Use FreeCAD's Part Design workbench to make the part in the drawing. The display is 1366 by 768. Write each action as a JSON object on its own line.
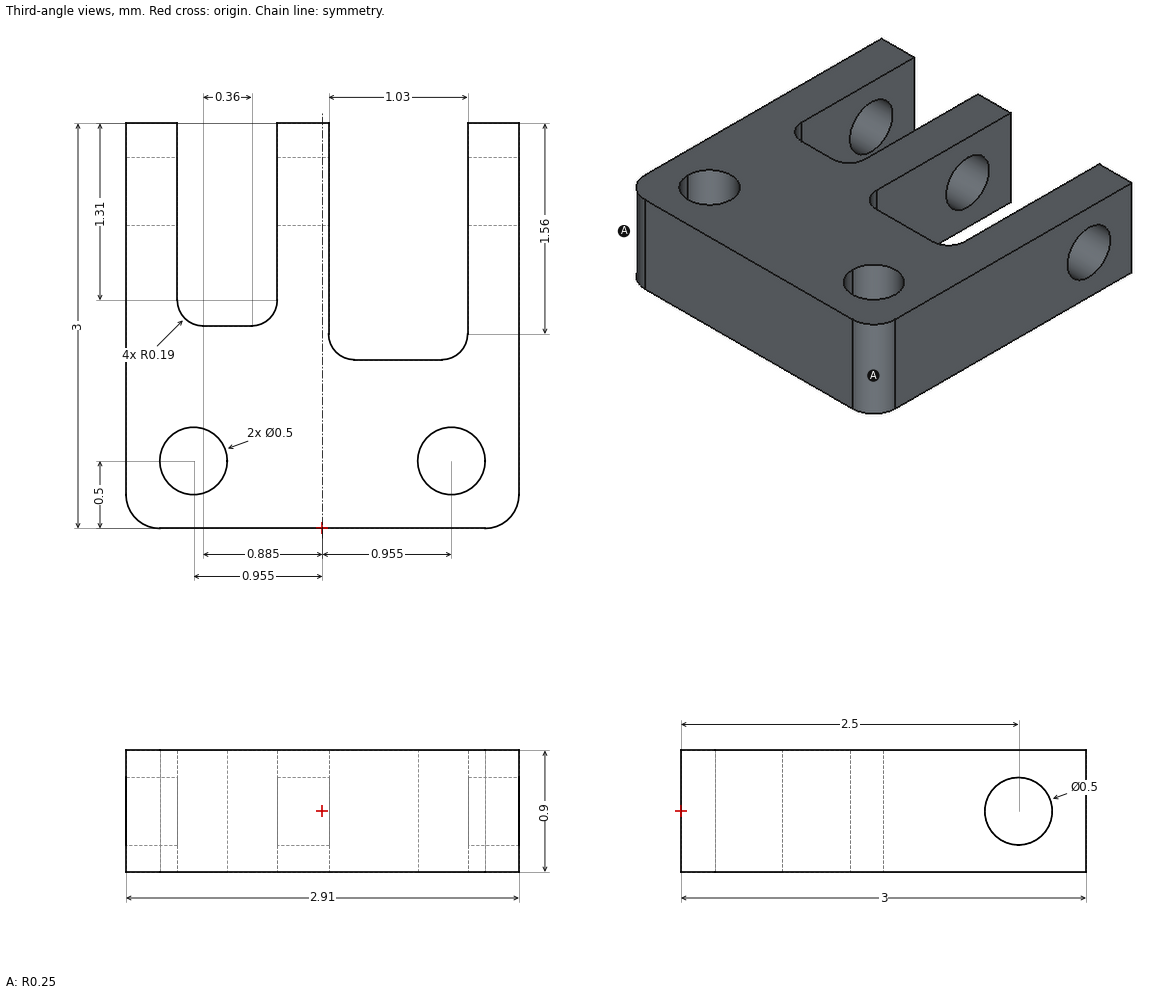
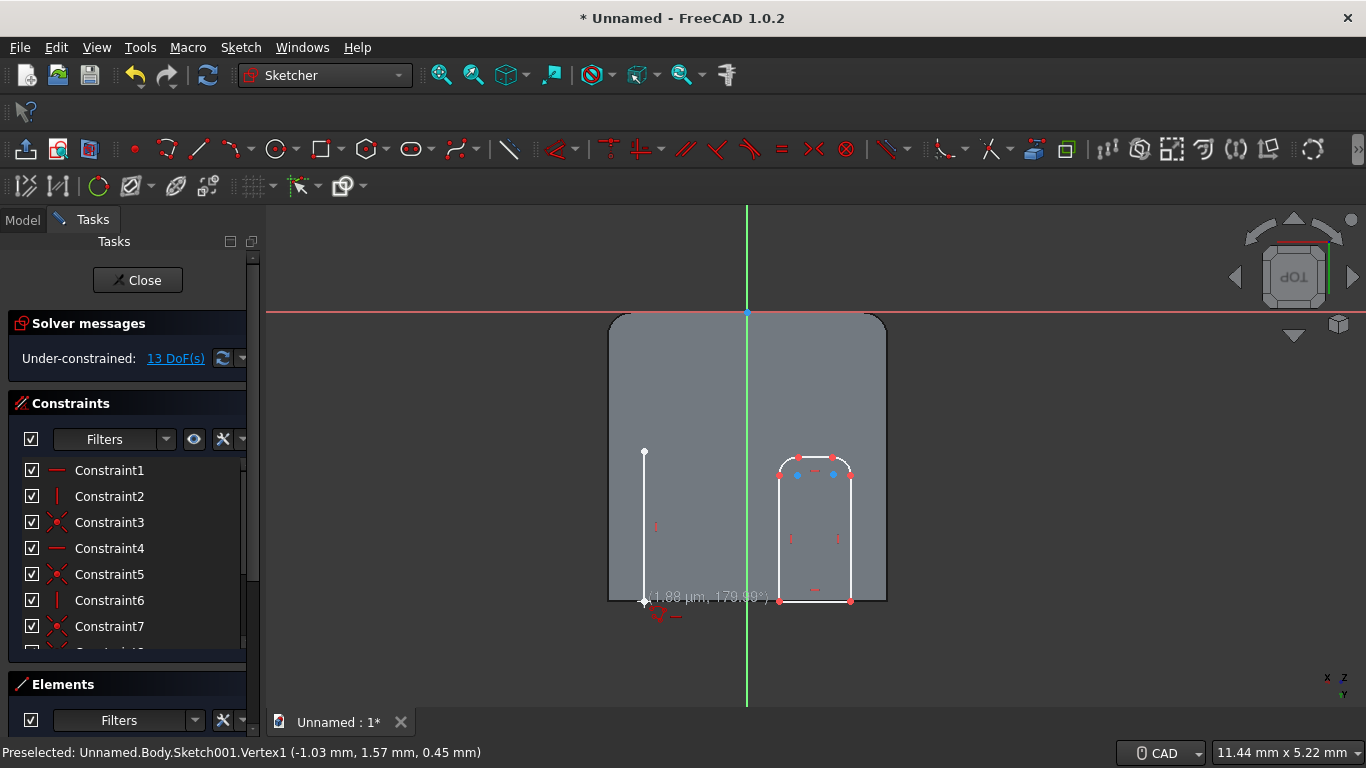
{"action": "scroll", "coordinate": [743, 601], "scroll_direction": "up", "scroll_amount": 7}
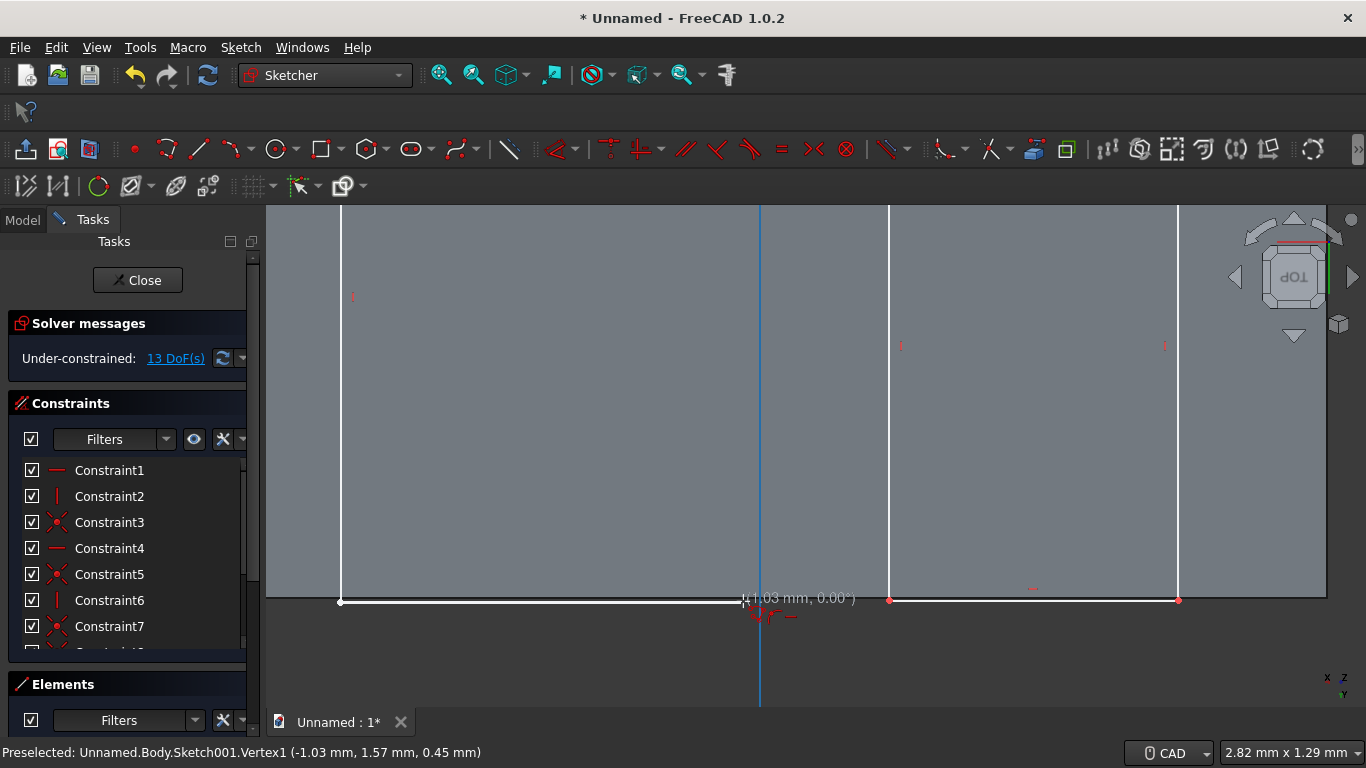
{"action": "left_click", "coordinate": [742, 599]}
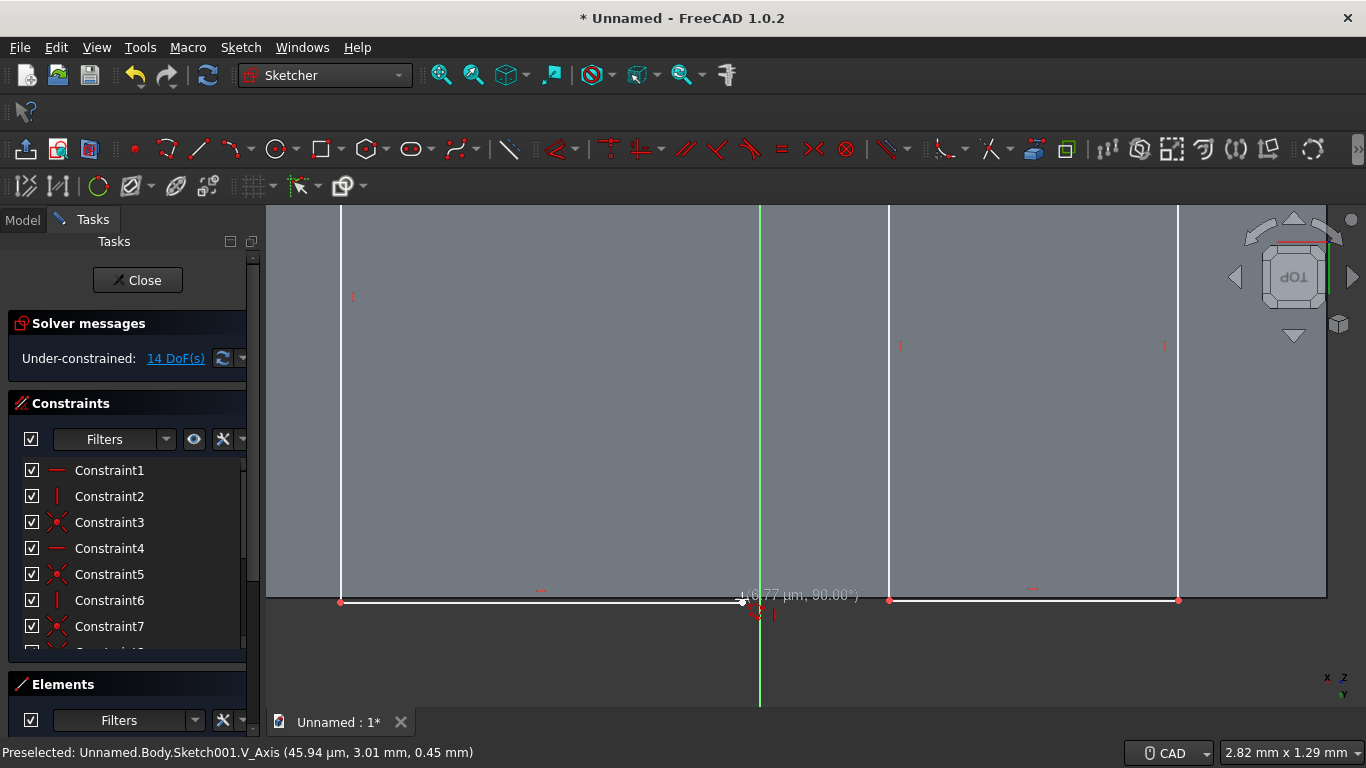
{"action": "scroll", "coordinate": [743, 601], "scroll_direction": "down", "scroll_amount": 7}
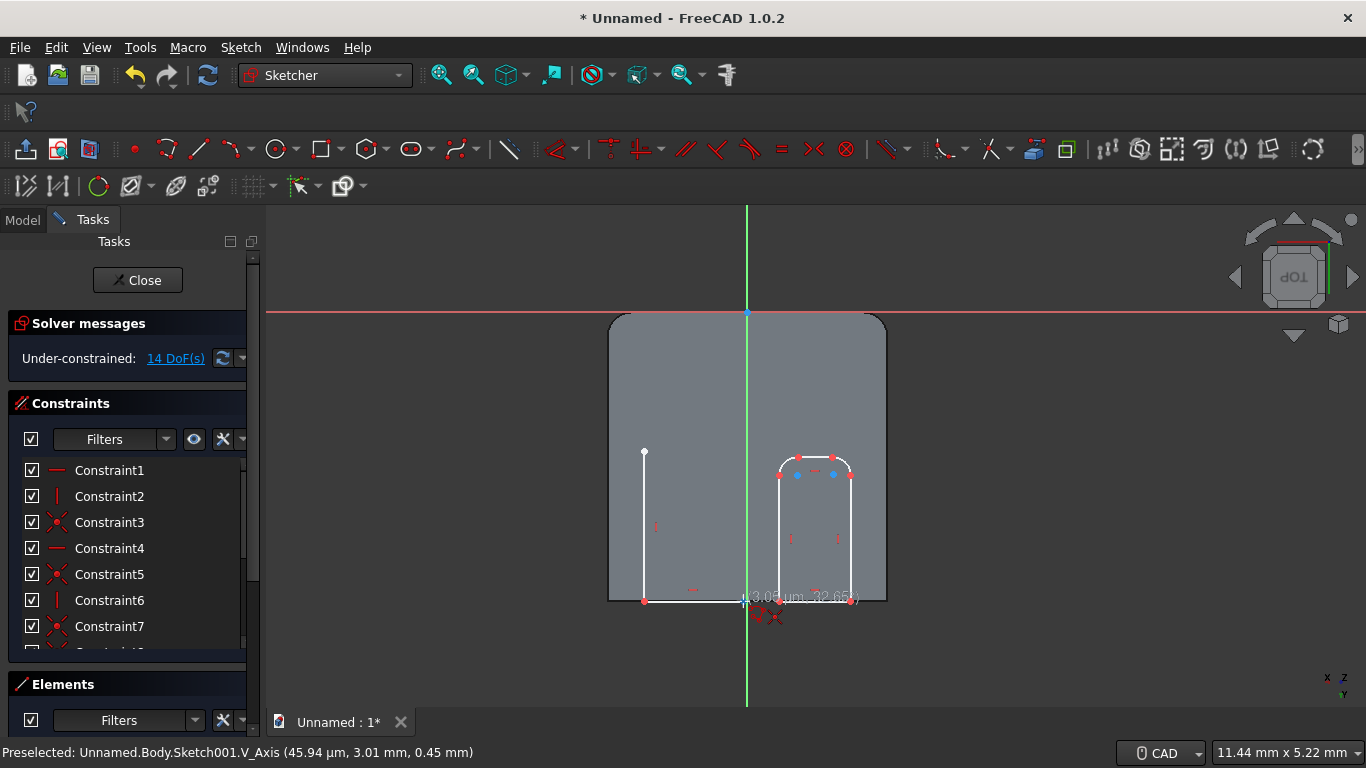
{"action": "scroll", "coordinate": [743, 451], "scroll_direction": "up", "scroll_amount": 7}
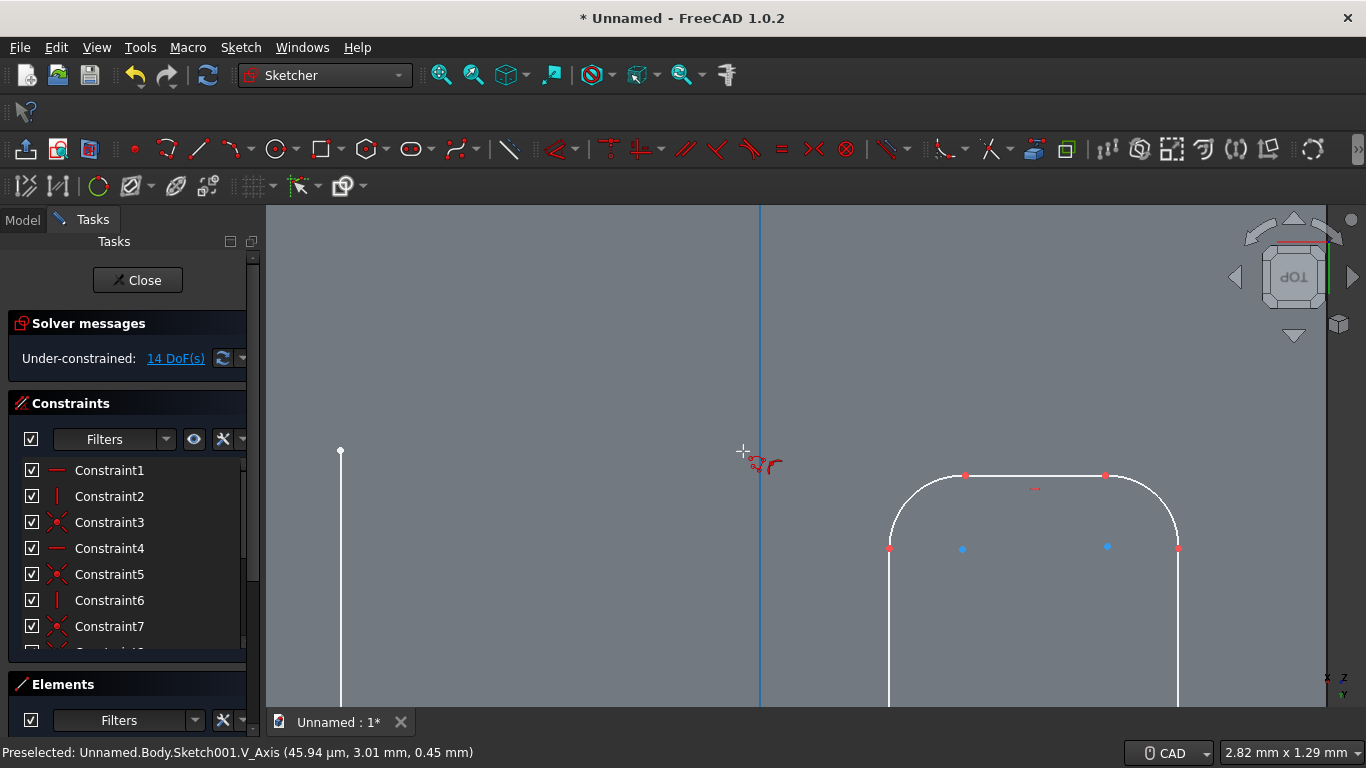
{"action": "left_click", "coordinate": [742, 449]}
{"action": "right_click", "coordinate": [742, 449]}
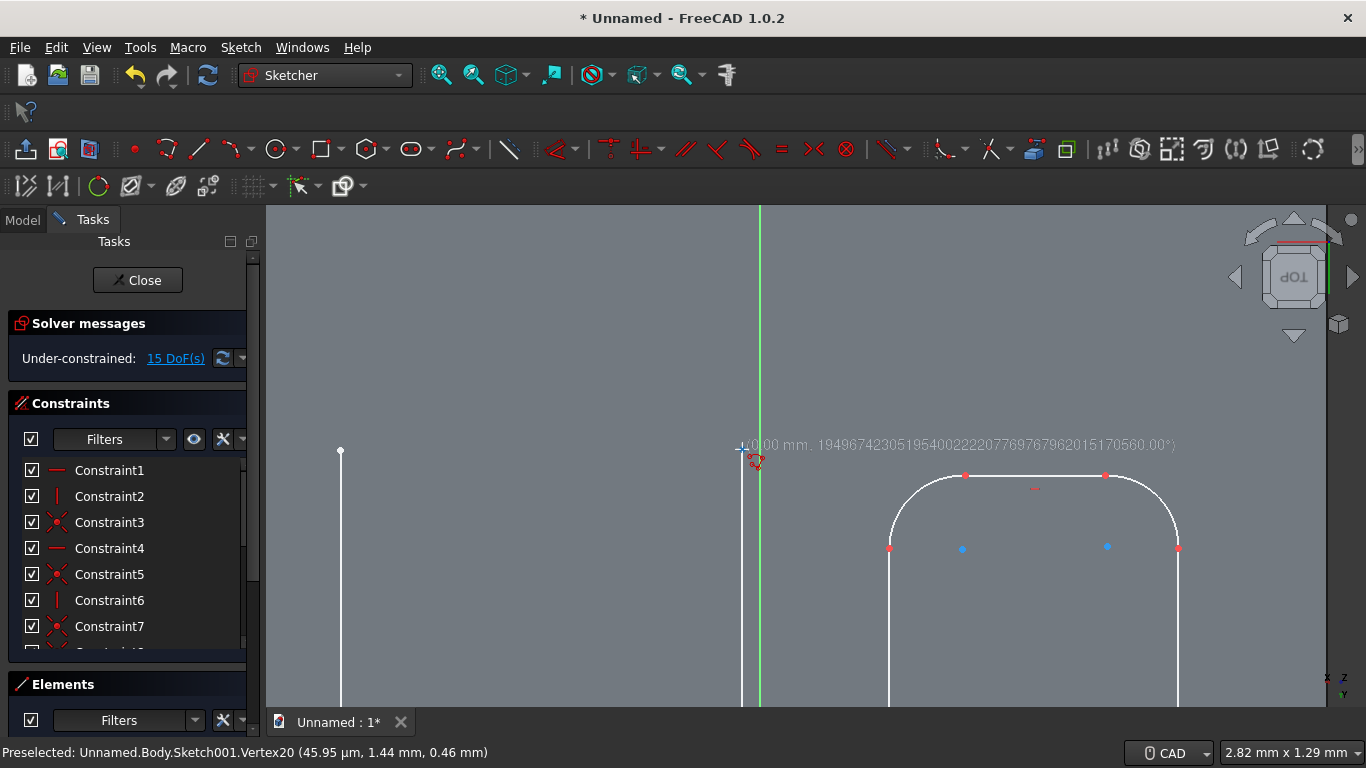
{"action": "key", "text": "g l"}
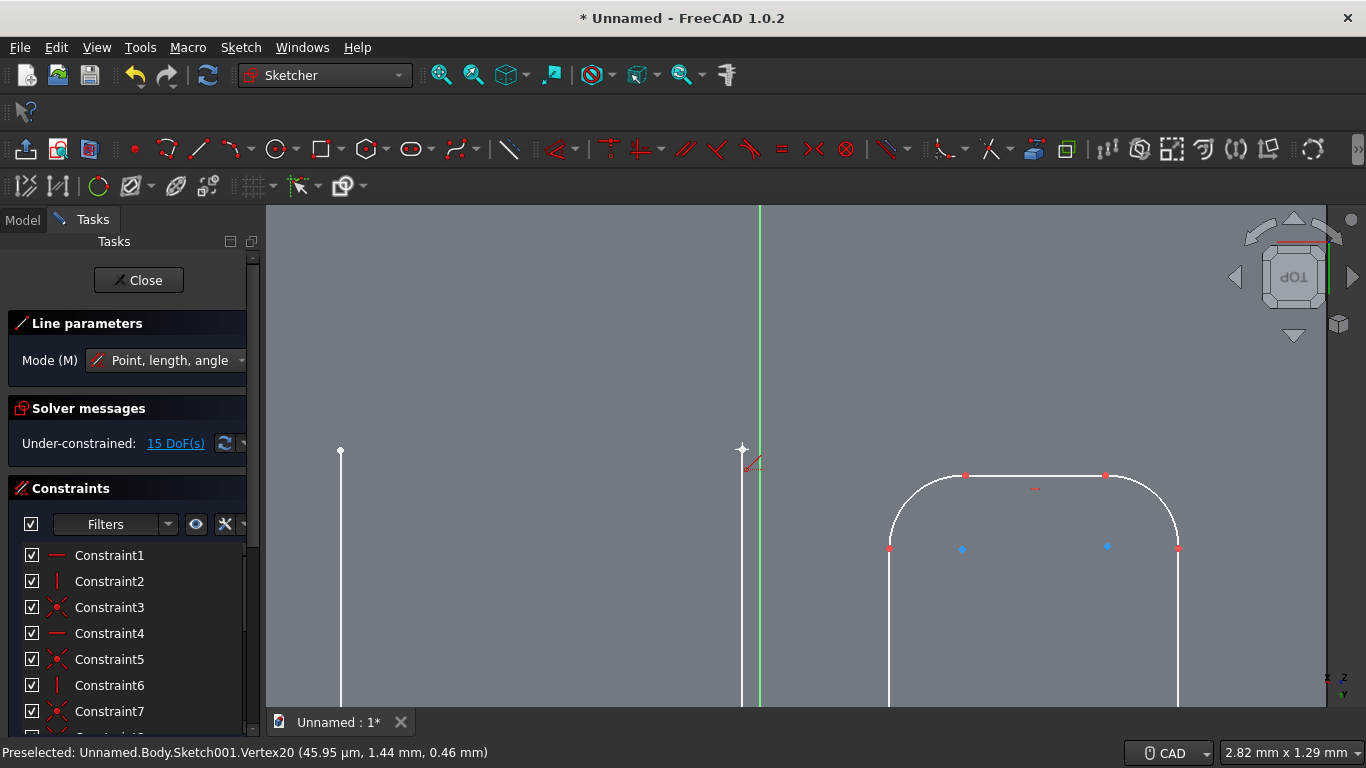
{"action": "left_click", "coordinate": [668, 375]}
{"action": "left_click", "coordinate": [415, 375]}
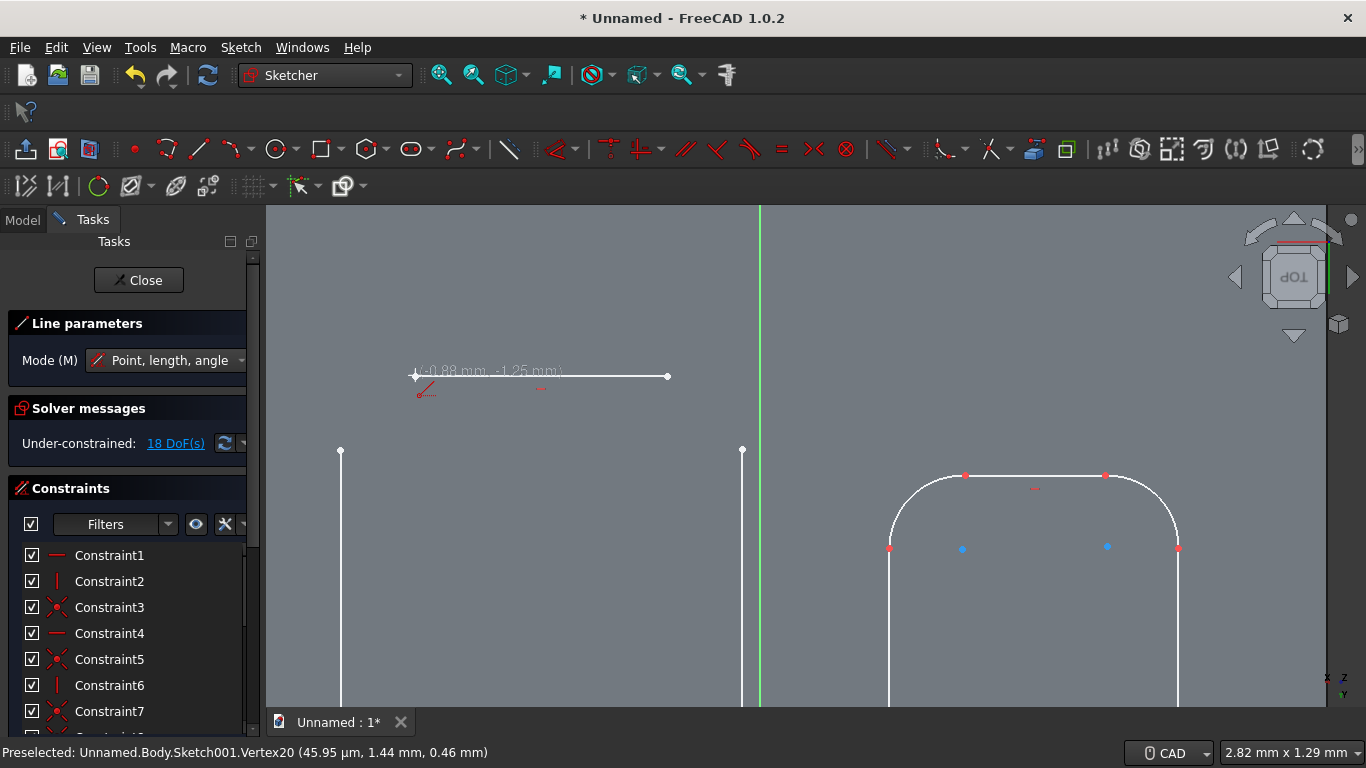
{"action": "key", "text": "g 3 a"}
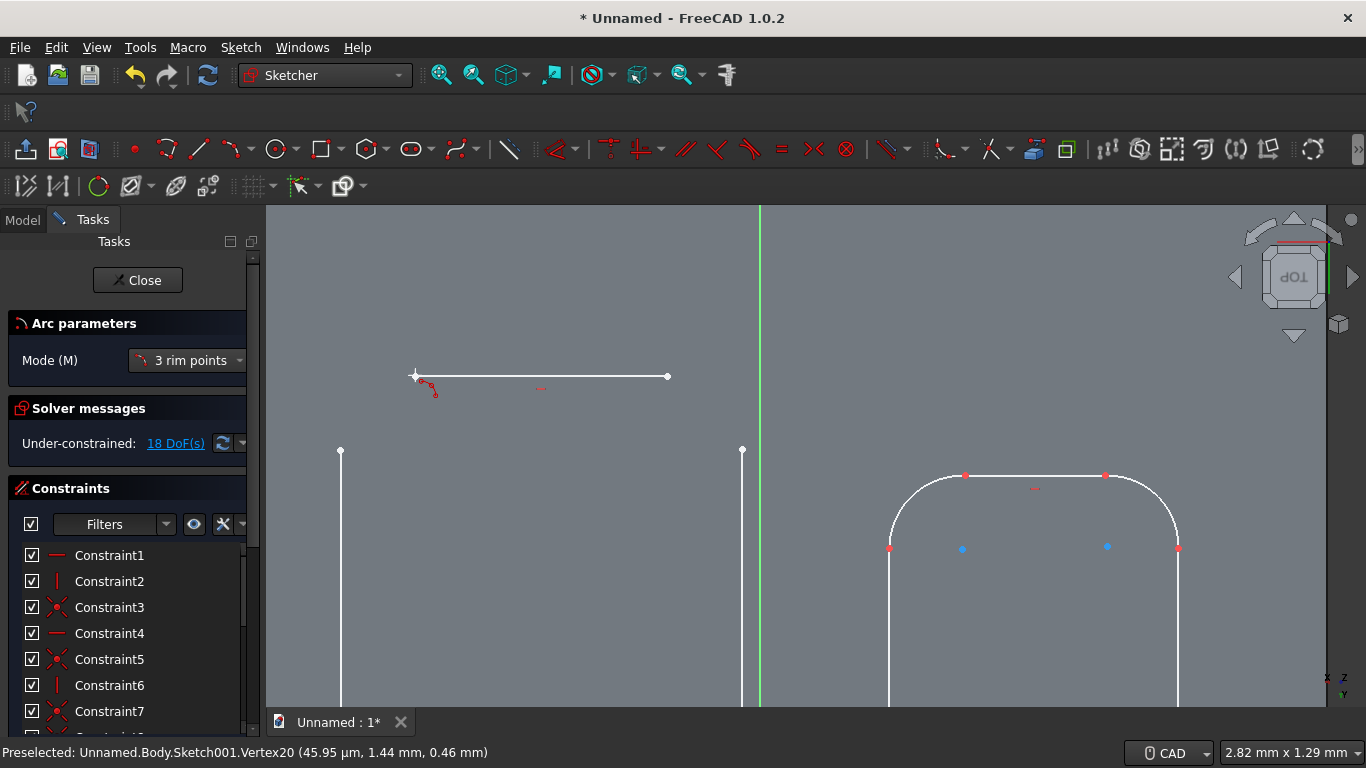
{"action": "left_click", "coordinate": [742, 450]}
{"action": "left_click", "coordinate": [668, 376]}
{"action": "left_click", "coordinate": [721, 397]}